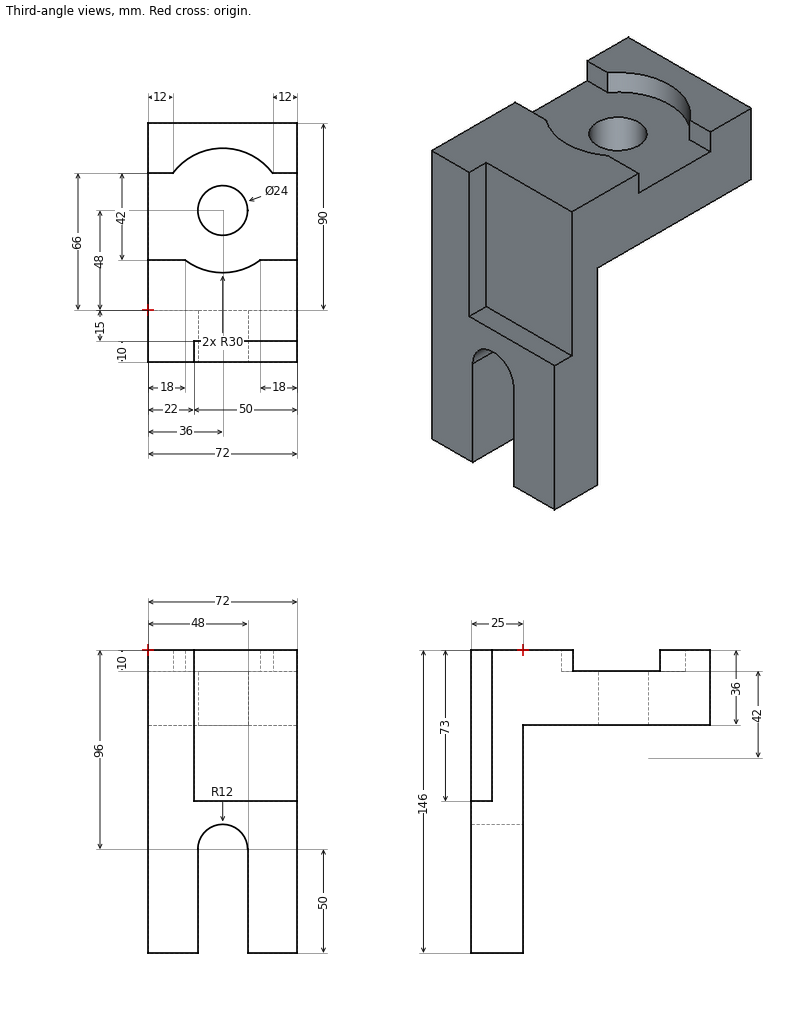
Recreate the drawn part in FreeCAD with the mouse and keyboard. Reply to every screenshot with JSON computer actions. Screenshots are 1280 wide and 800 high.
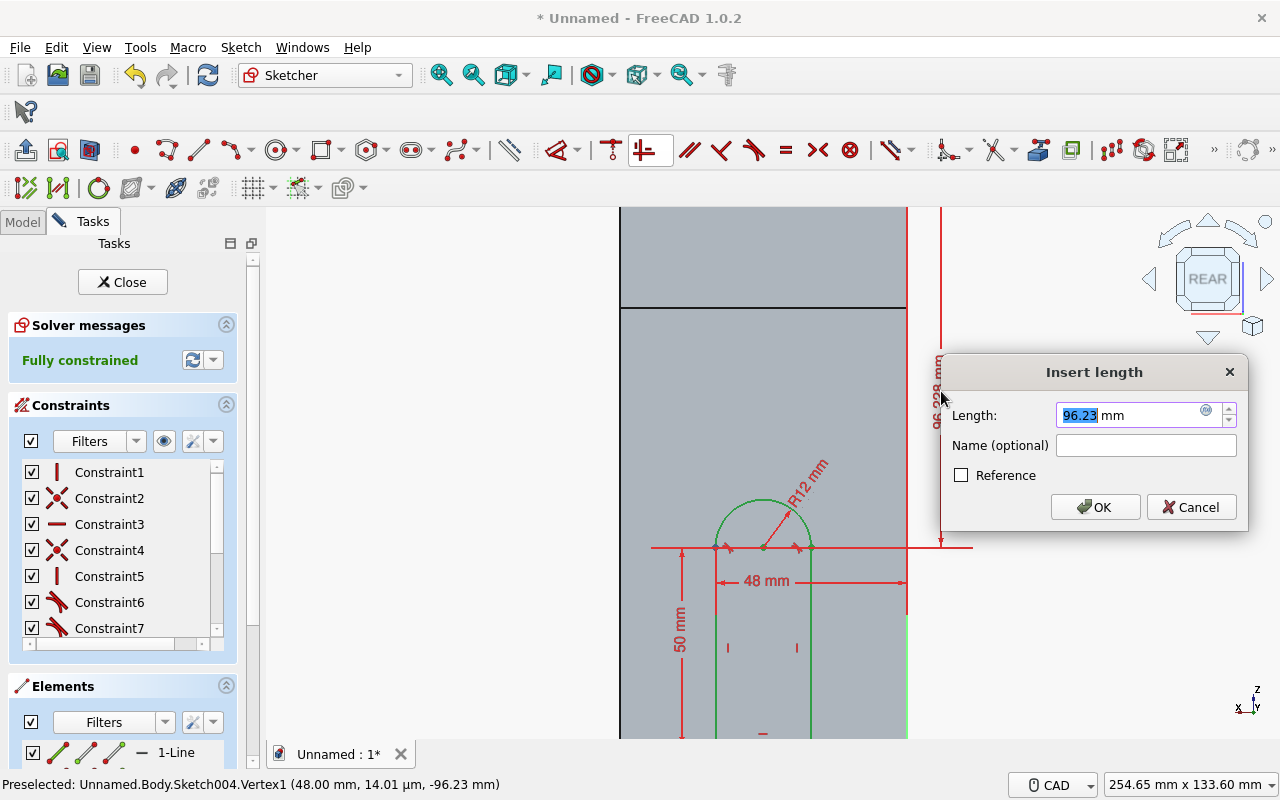
{"action": "type", "text": "96"}
{"action": "key", "text": "Return"}
{"action": "key", "text": "Escape"}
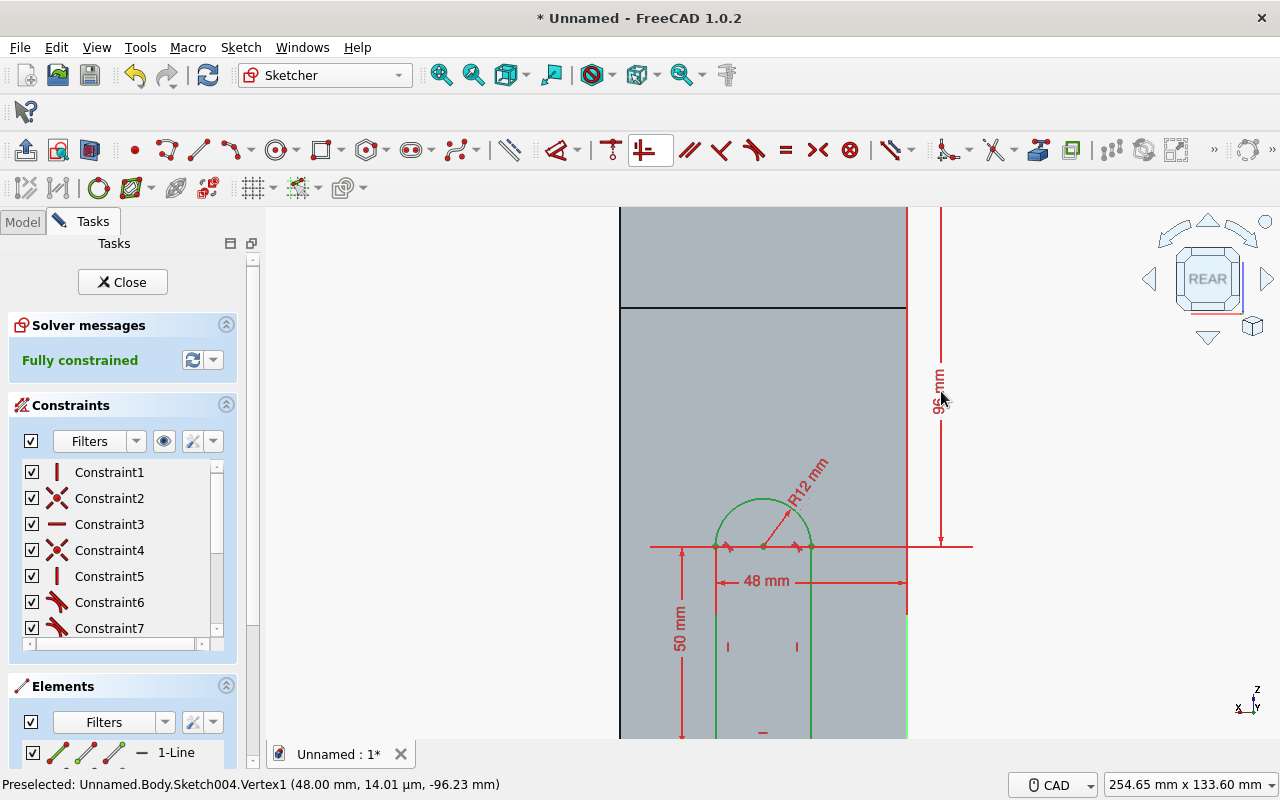
{"action": "left_click", "coordinate": [123, 282]}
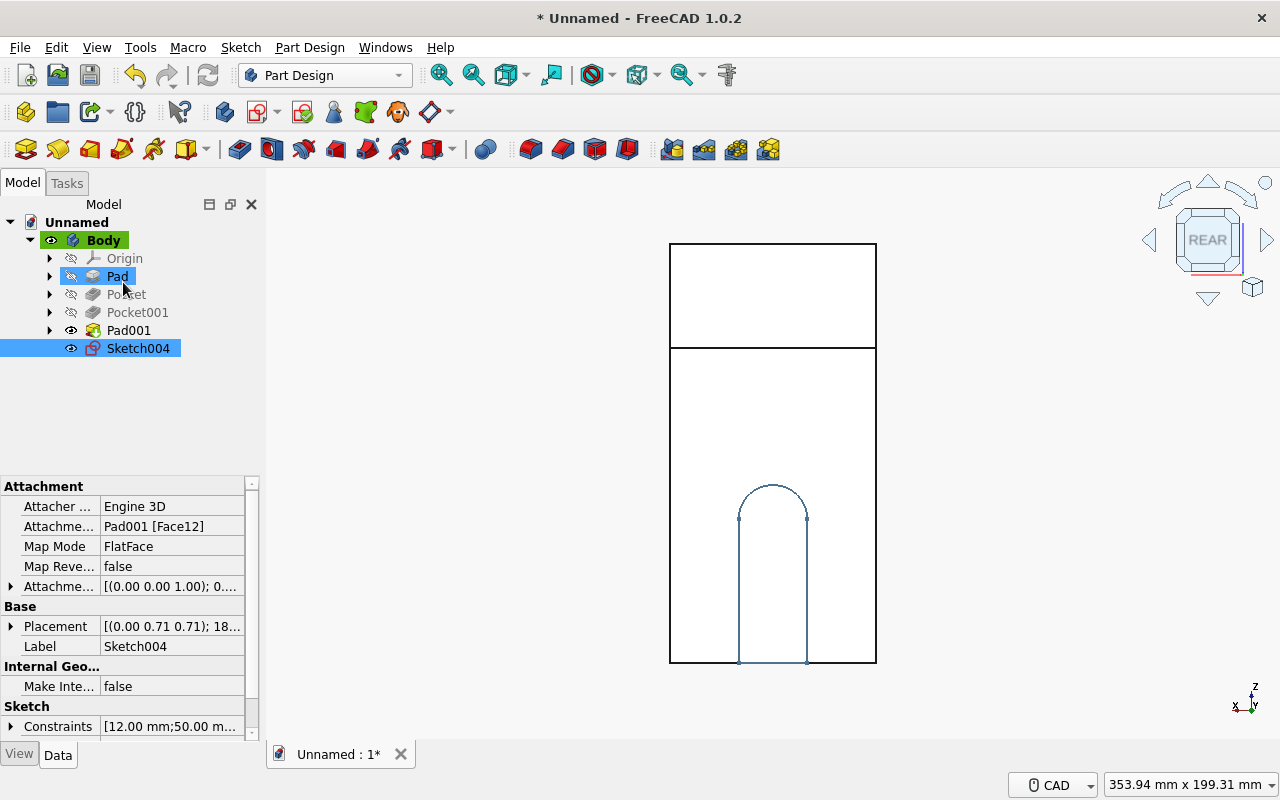
{"action": "left_click", "coordinate": [240, 150]}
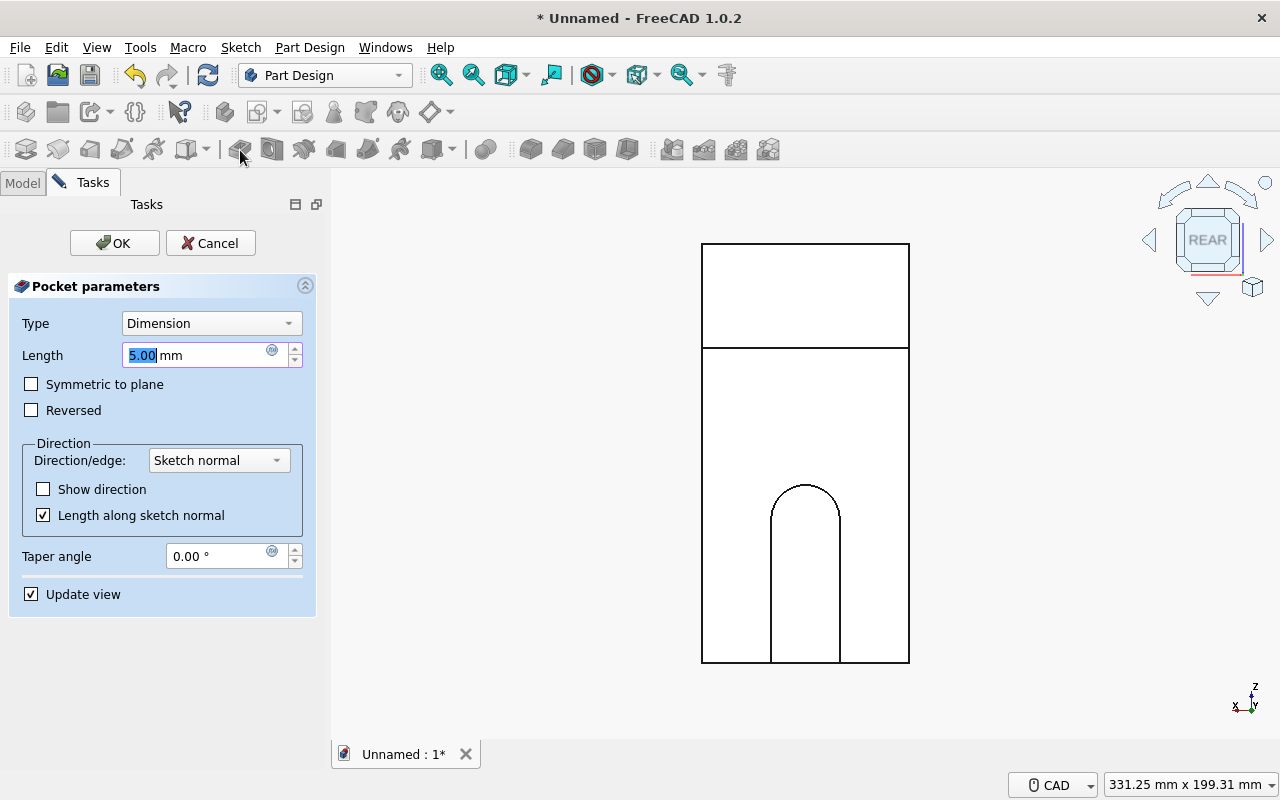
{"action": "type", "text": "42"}
{"action": "key", "text": "Tab"}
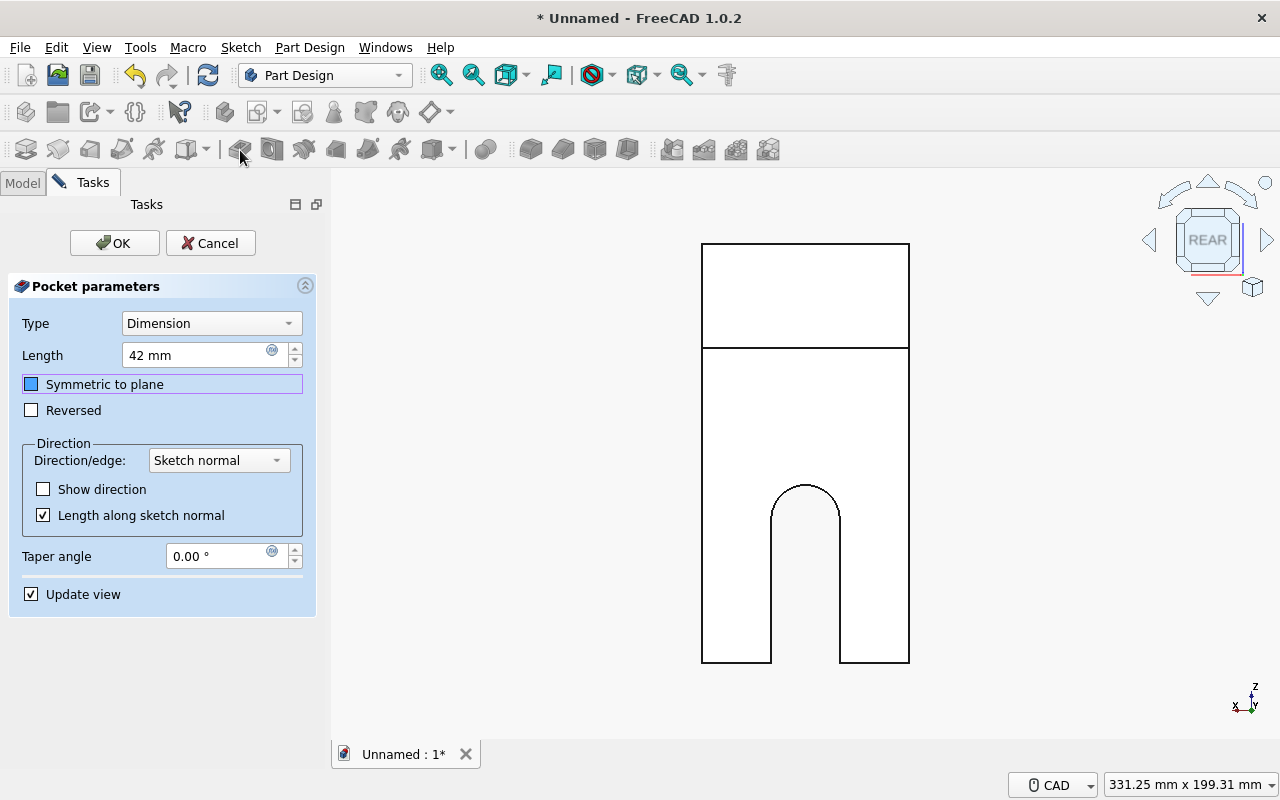
{"action": "left_click", "coordinate": [115, 243]}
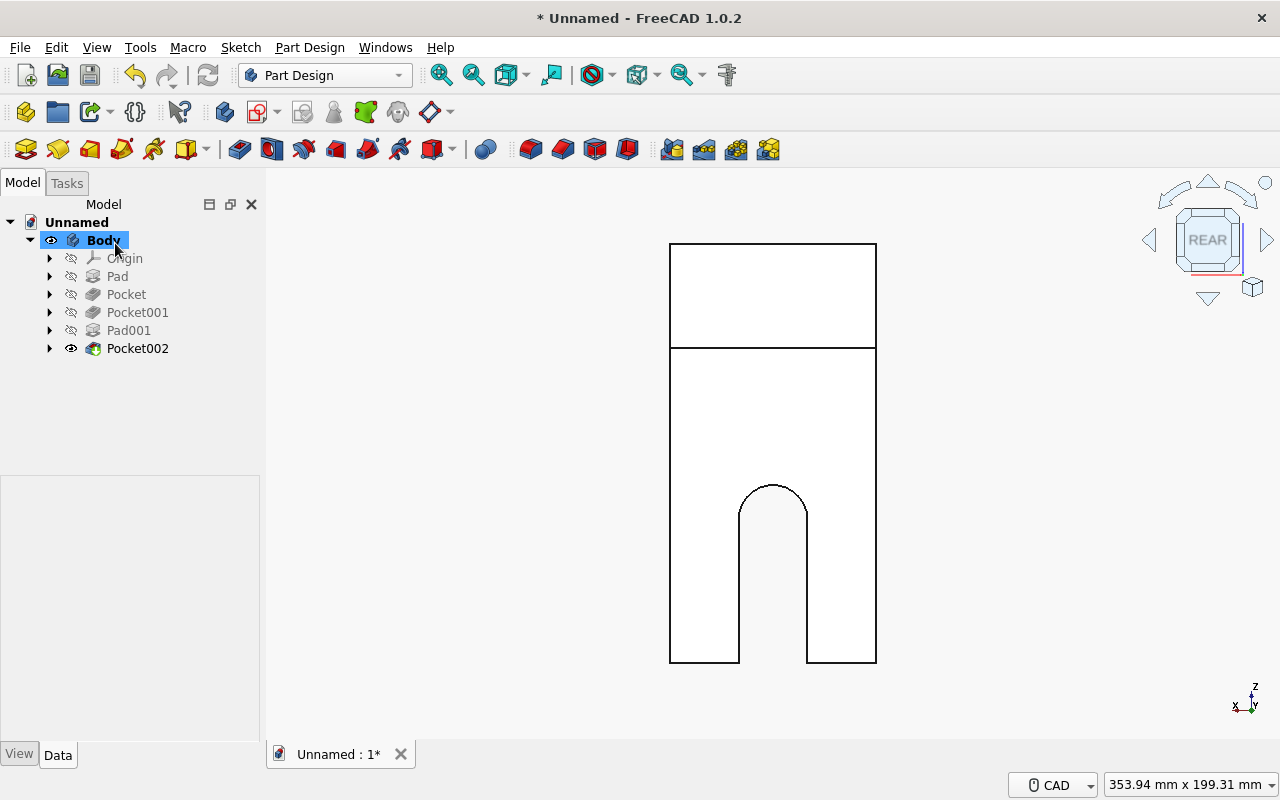
{"action": "left_click", "coordinate": [258, 112]}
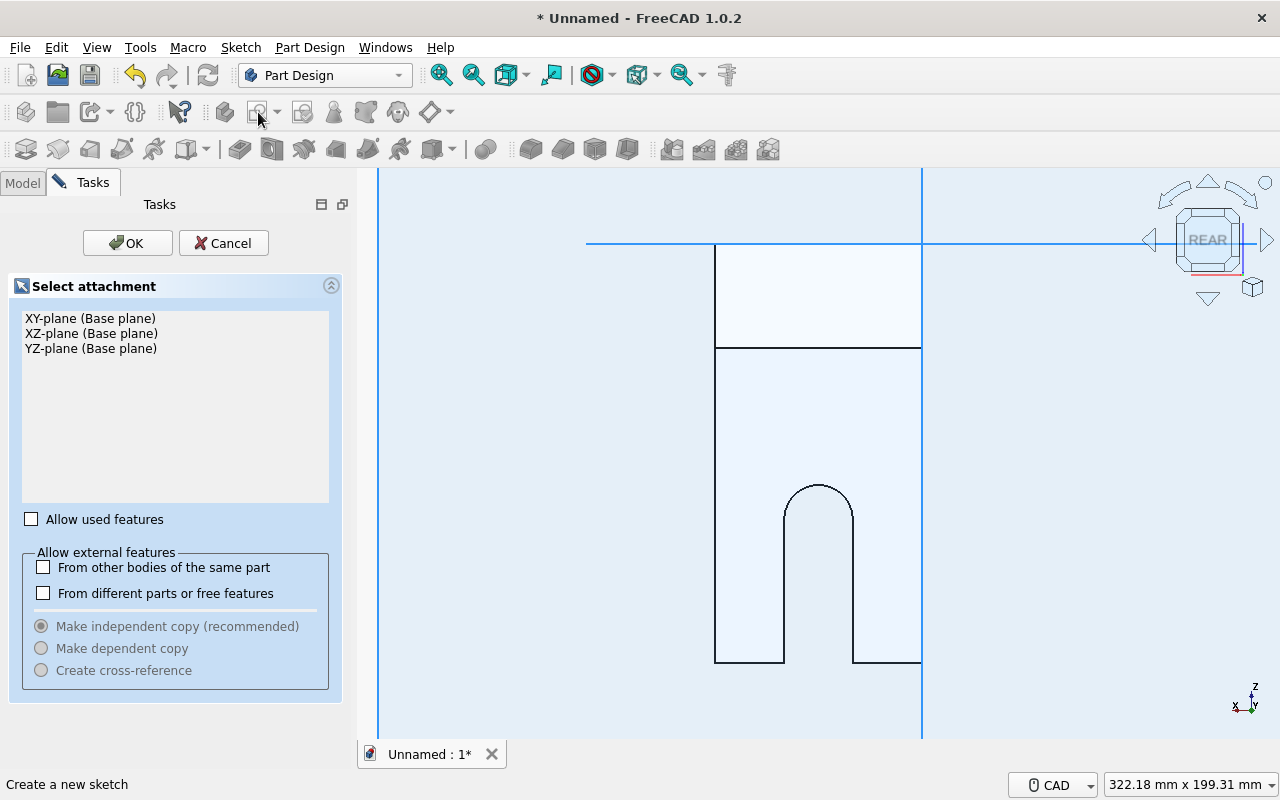
{"action": "left_click", "coordinate": [82, 318]}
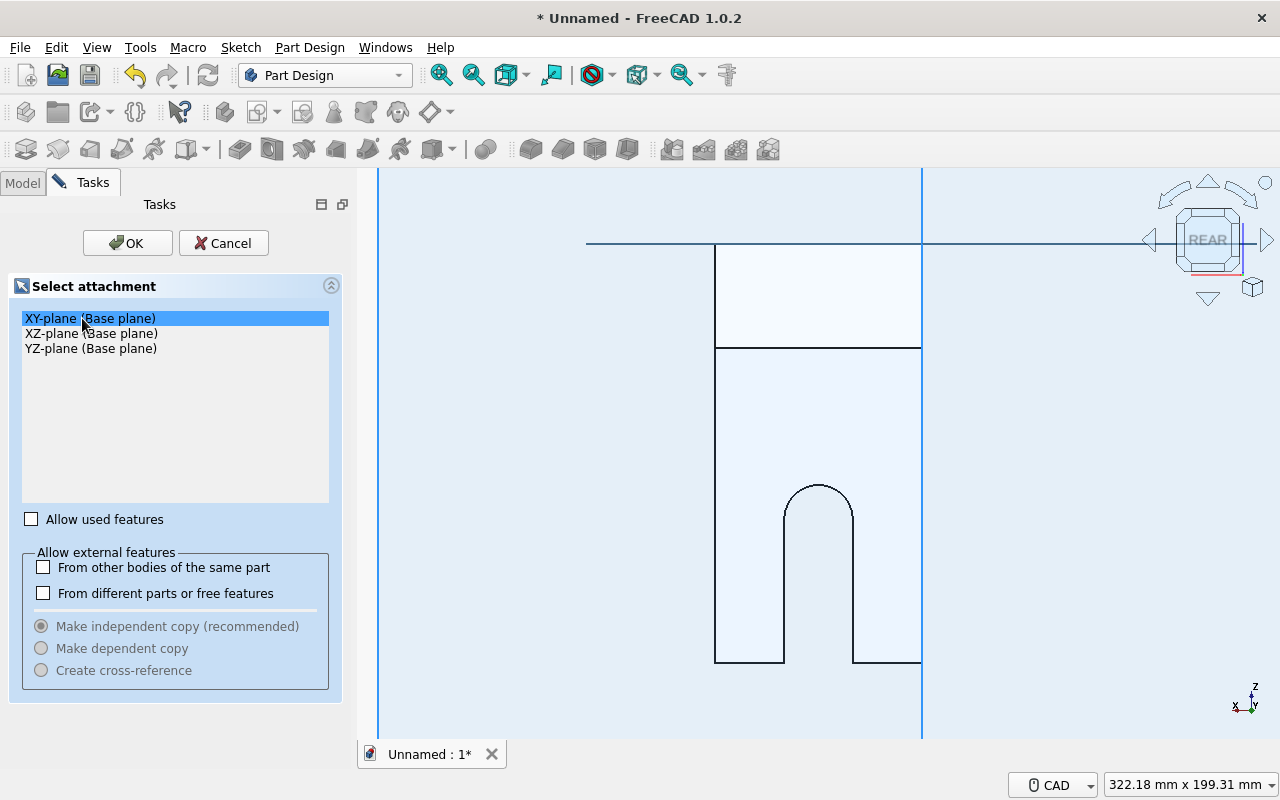
{"action": "left_click", "coordinate": [128, 243]}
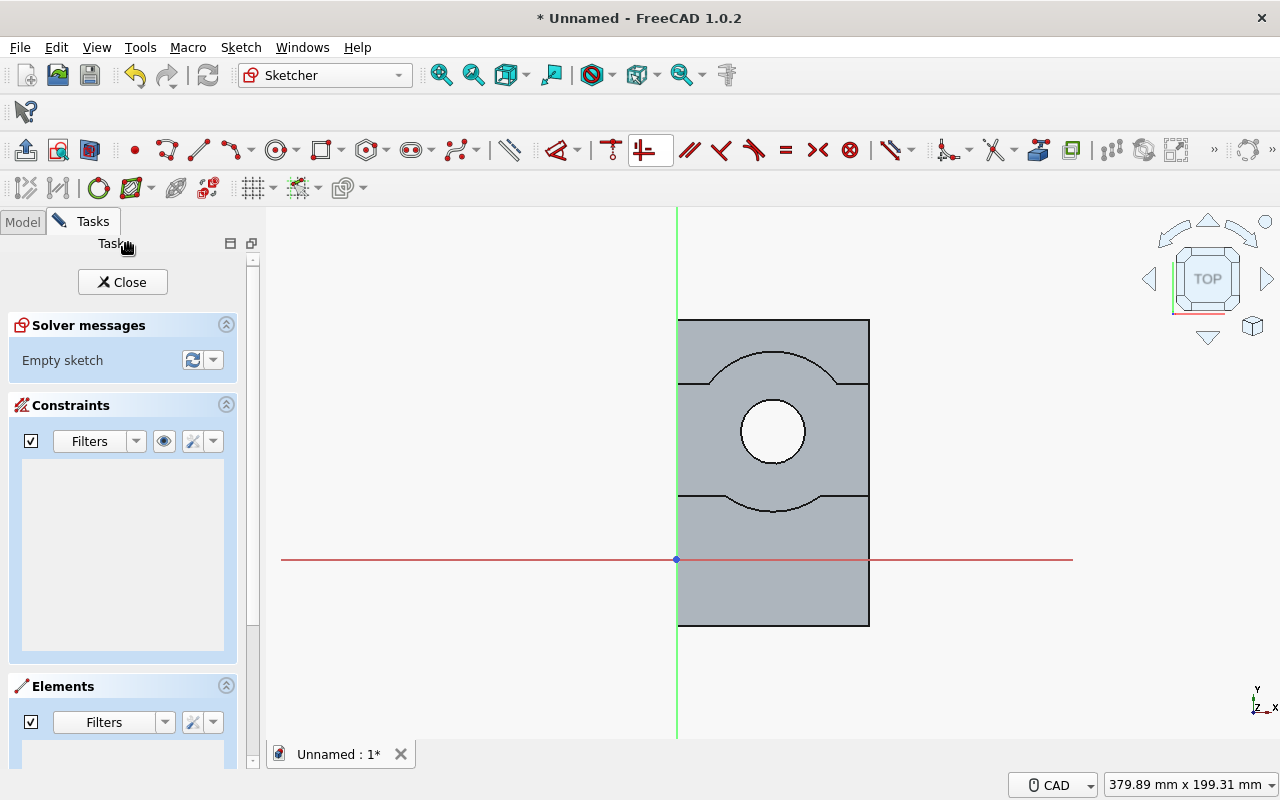
{"action": "scroll", "coordinate": [803, 645], "scroll_direction": "up", "scroll_amount": 6}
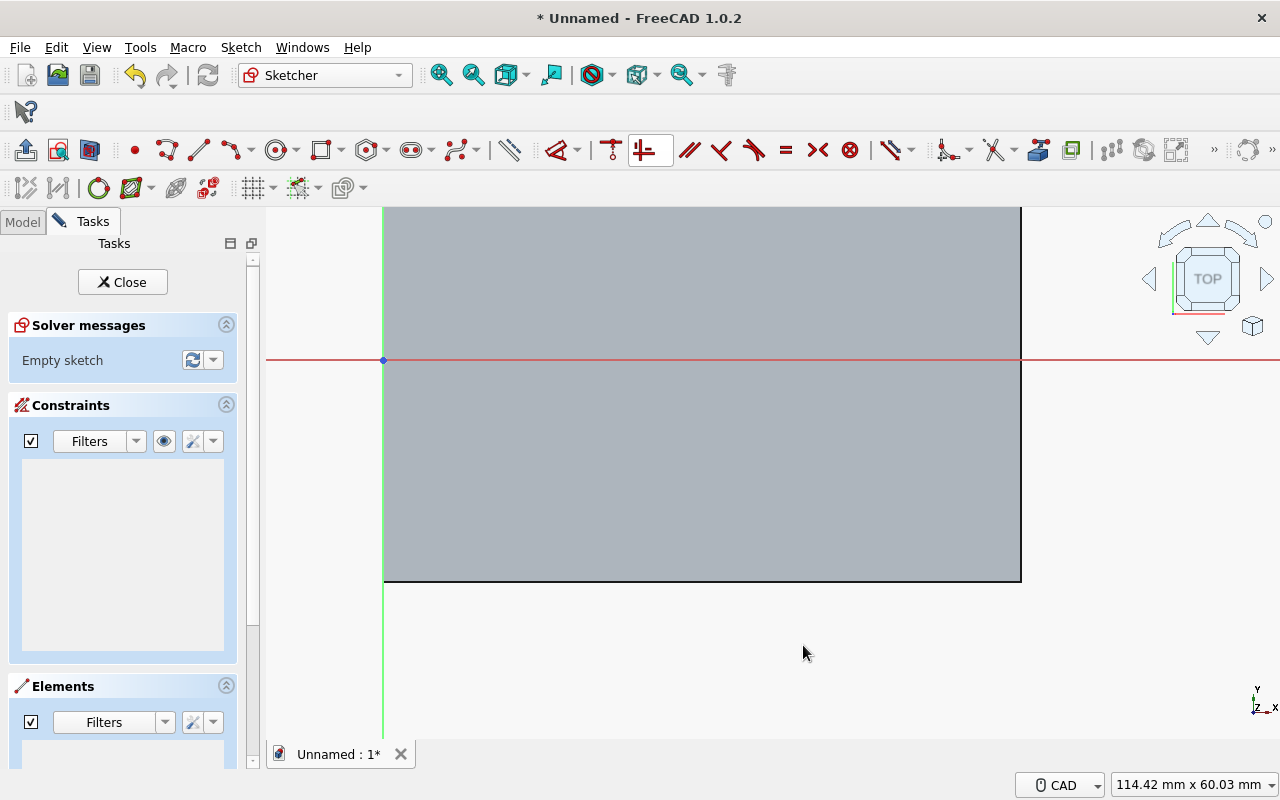
{"action": "left_click", "coordinate": [322, 150]}